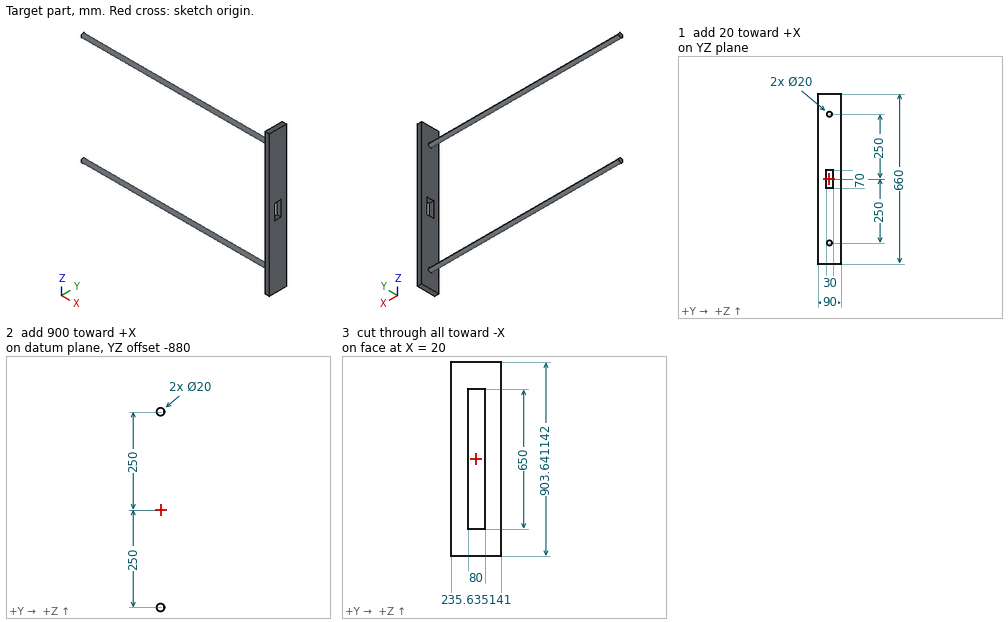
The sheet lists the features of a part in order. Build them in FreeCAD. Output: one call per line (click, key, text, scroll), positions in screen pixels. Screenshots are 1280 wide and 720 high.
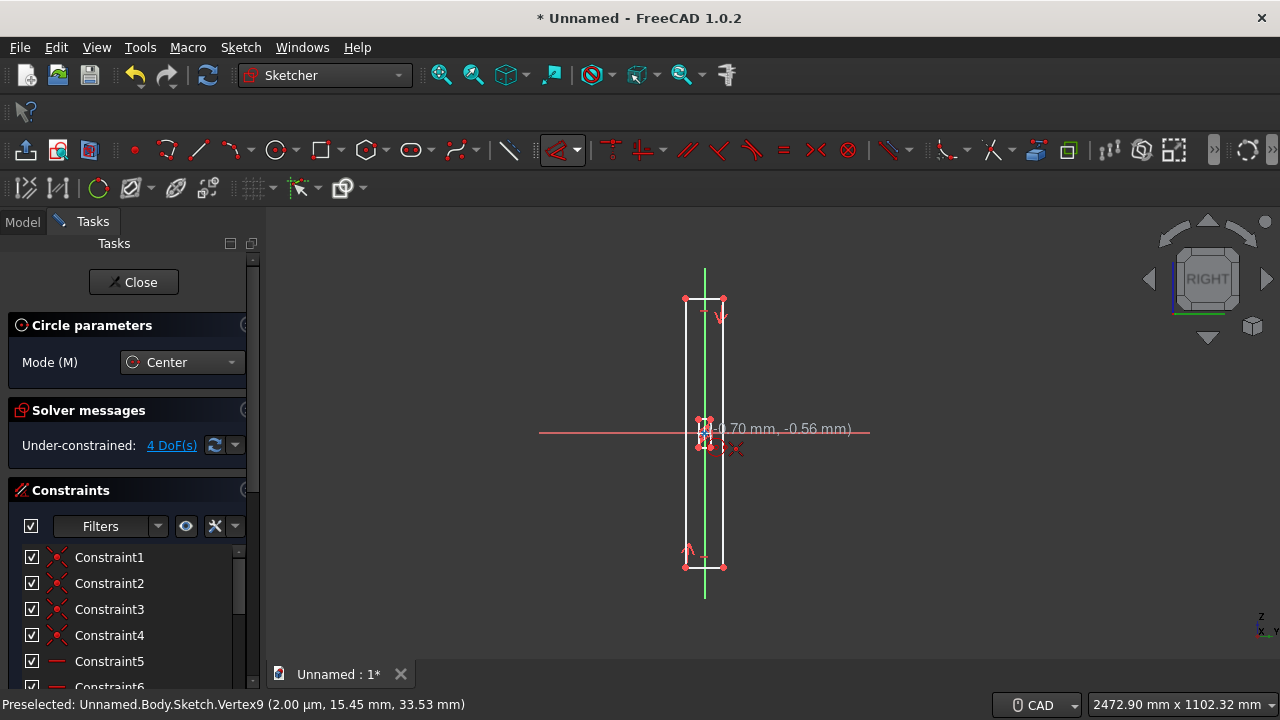
scroll(705, 331, up, 9)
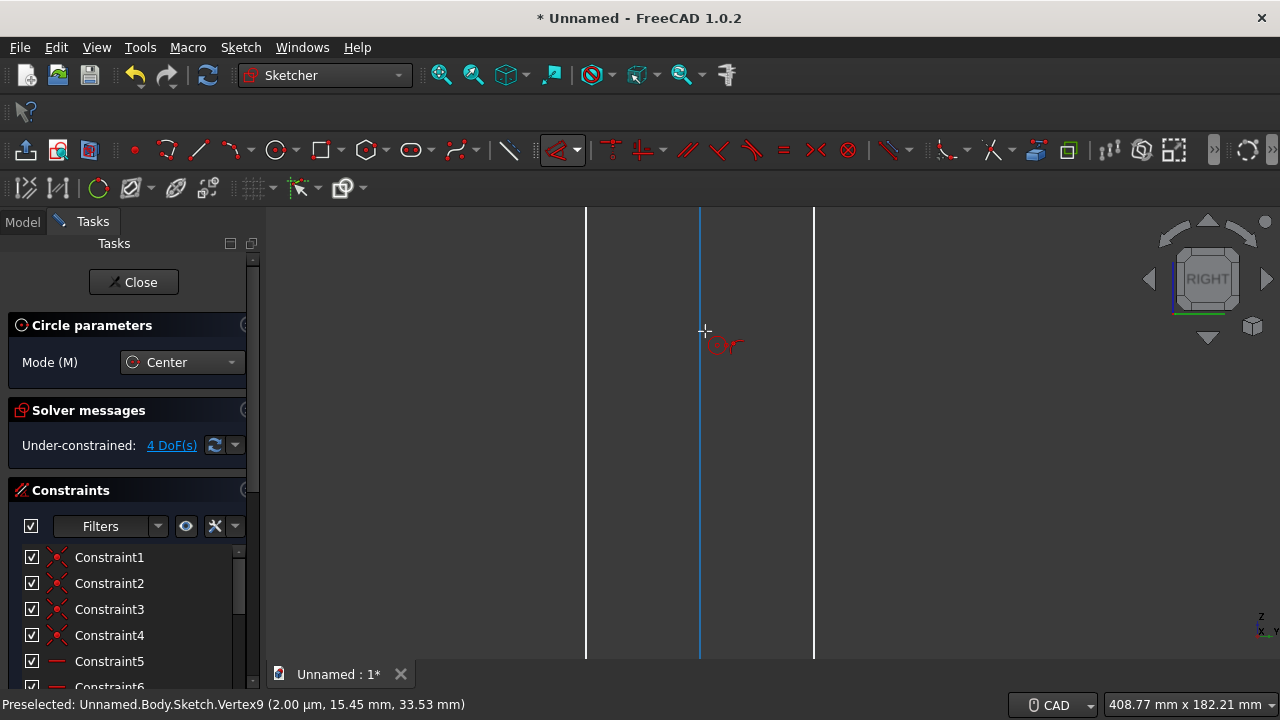
scroll(705, 331, down, 9)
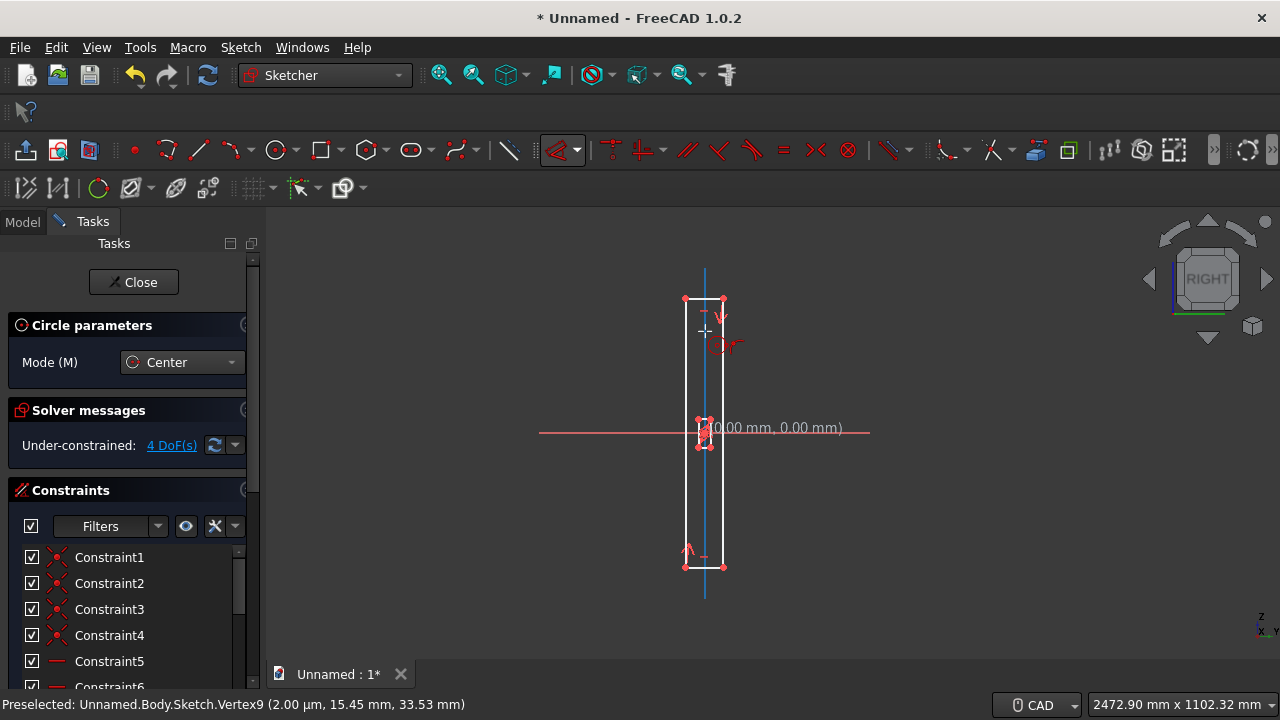
click(705, 331)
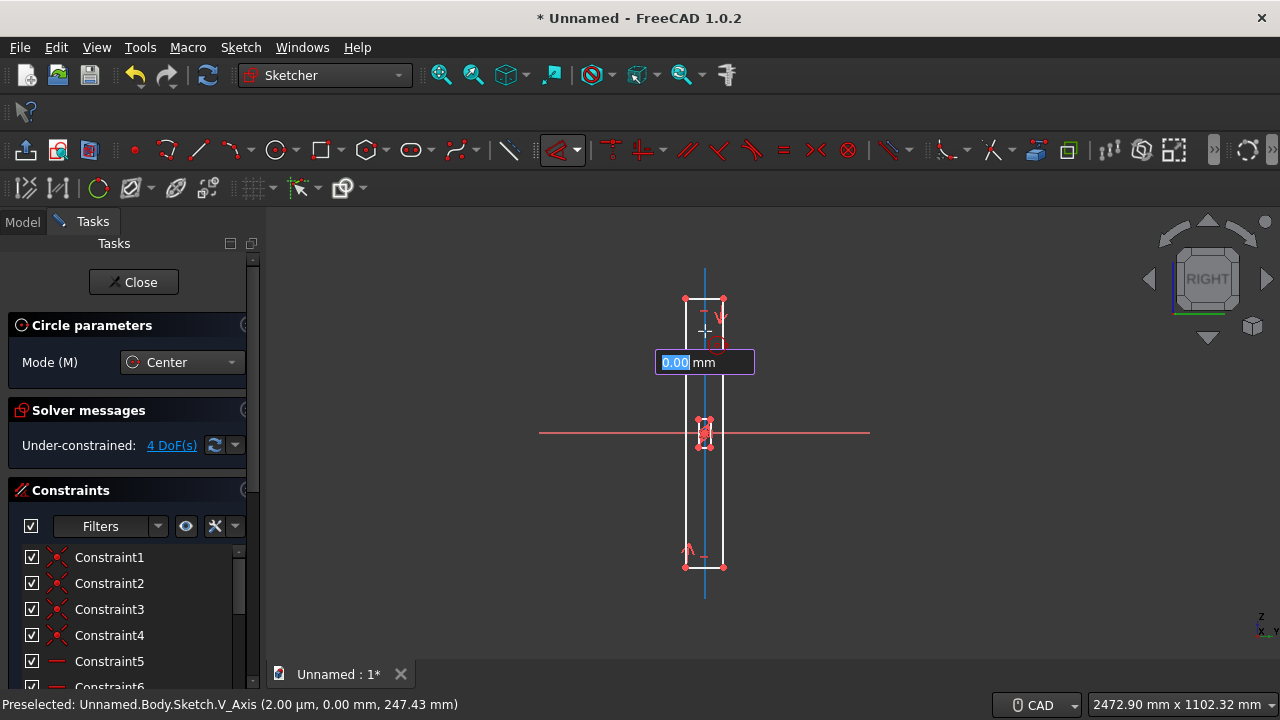
scroll(708, 330, up, 8)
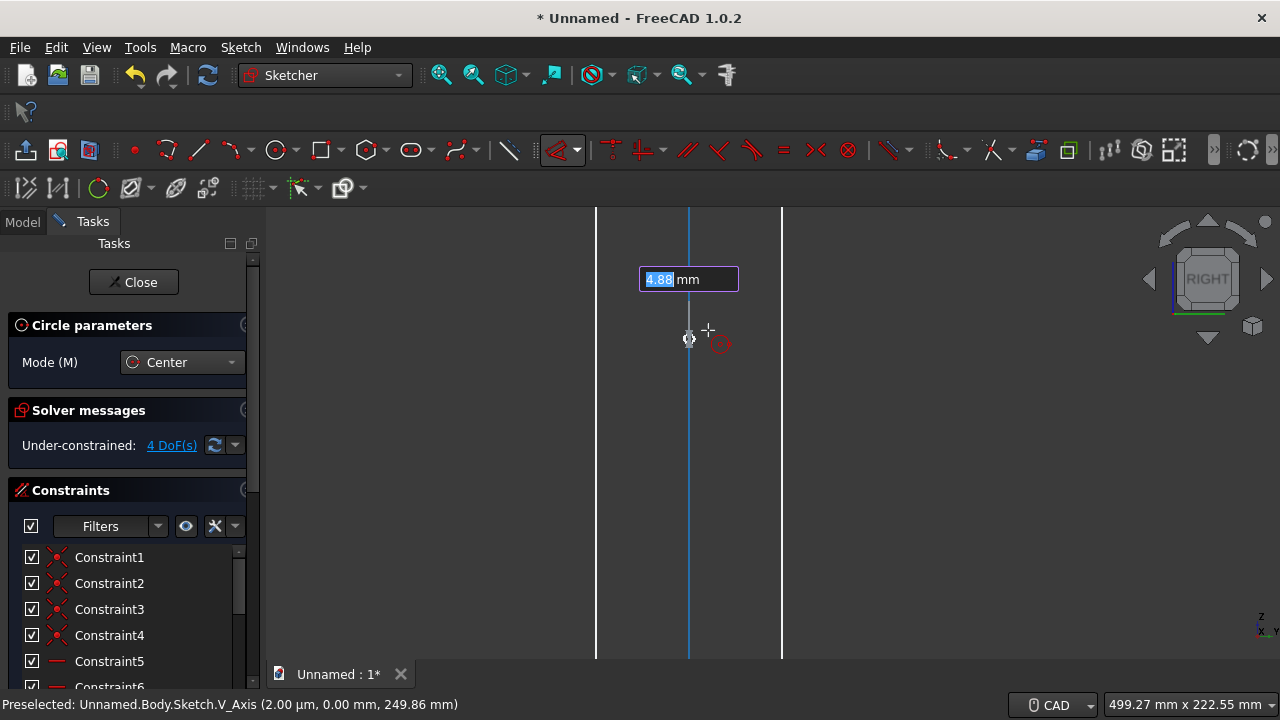
click(708, 327)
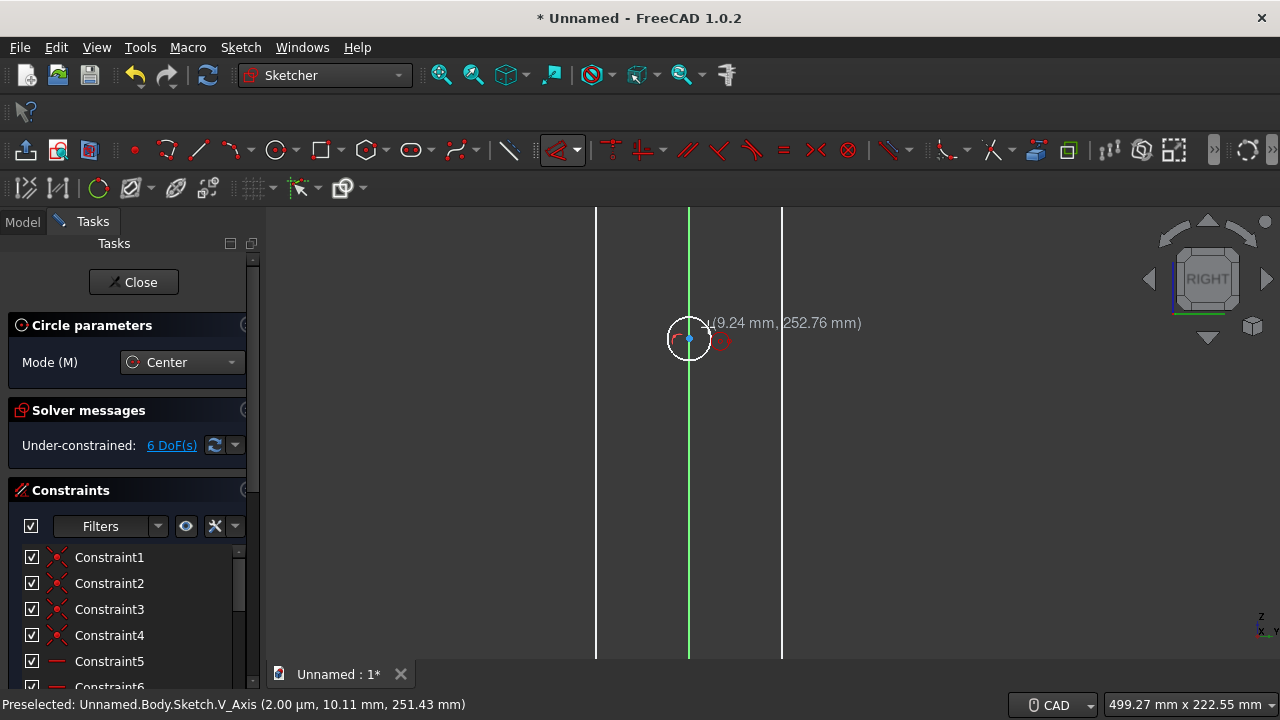
scroll(708, 330, down, 8)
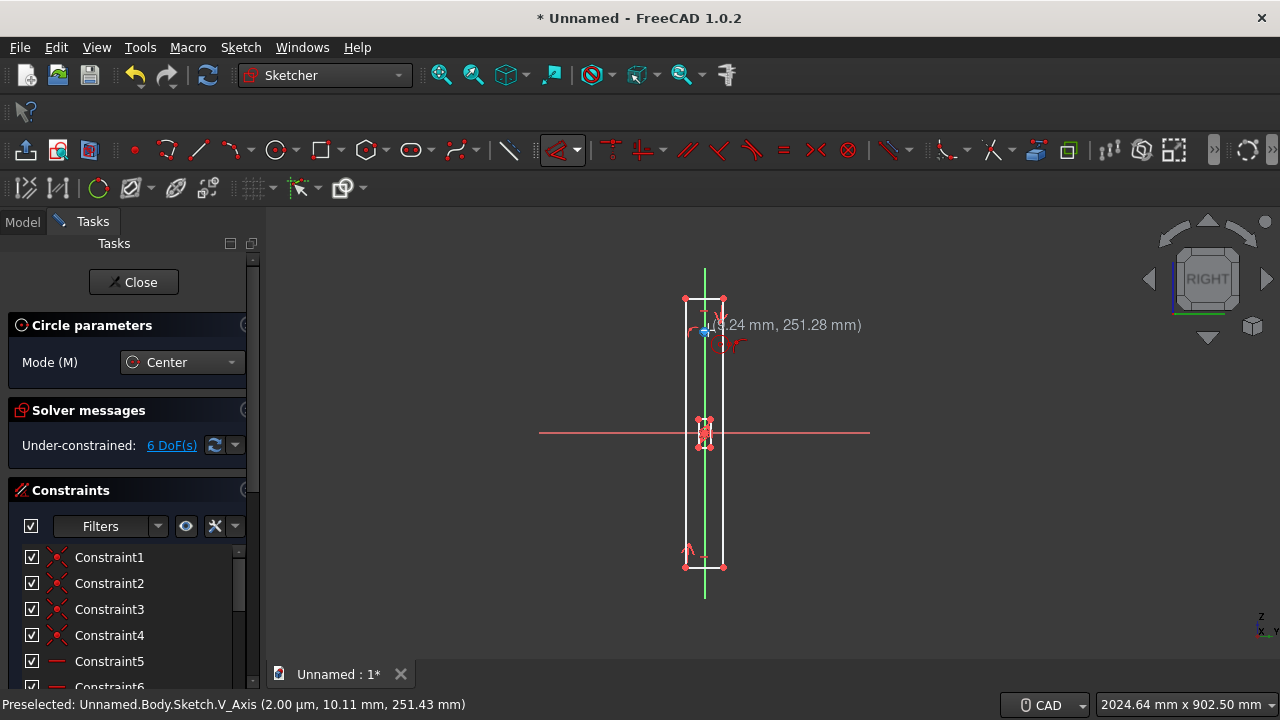
scroll(705, 536, up, 9)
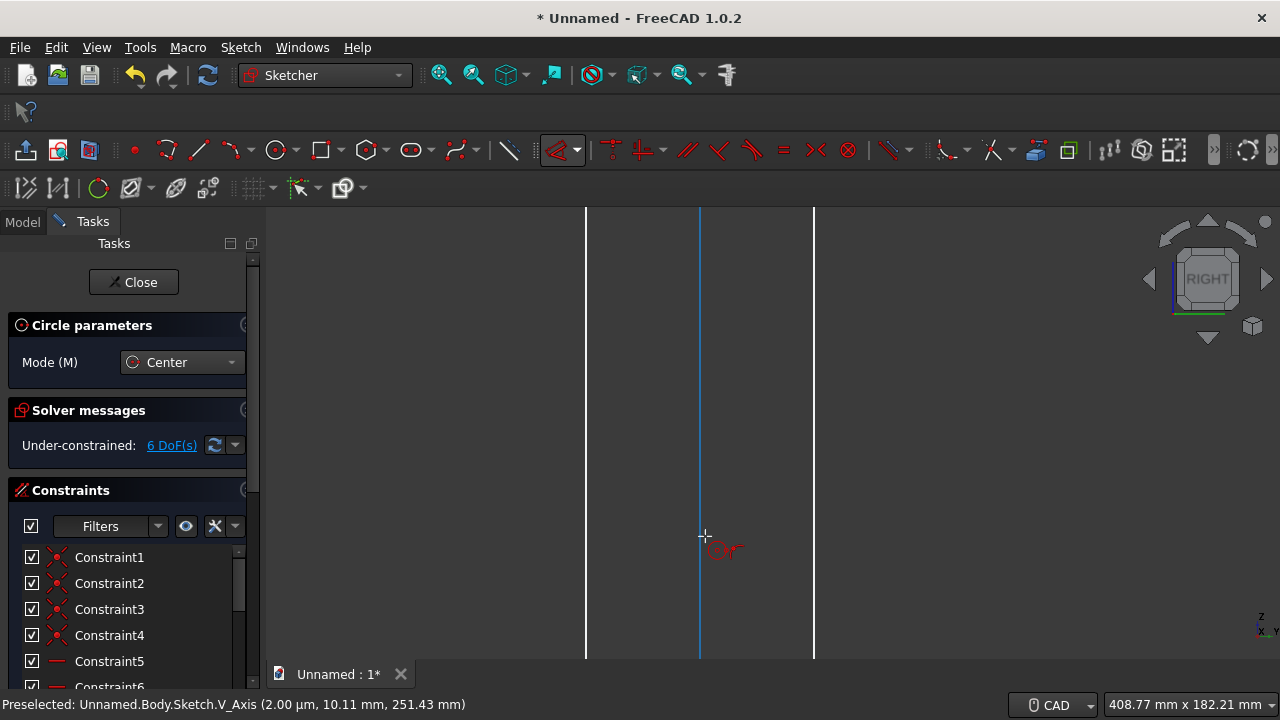
scroll(705, 536, down, 9)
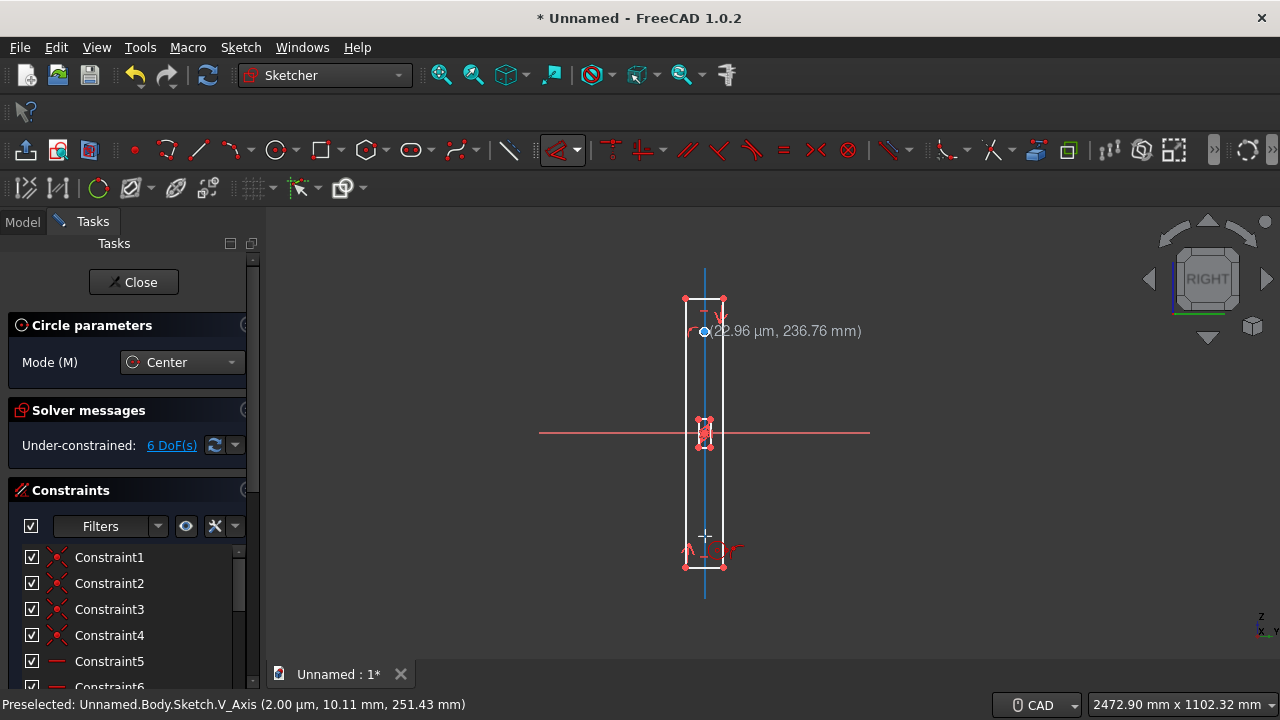
click(705, 536)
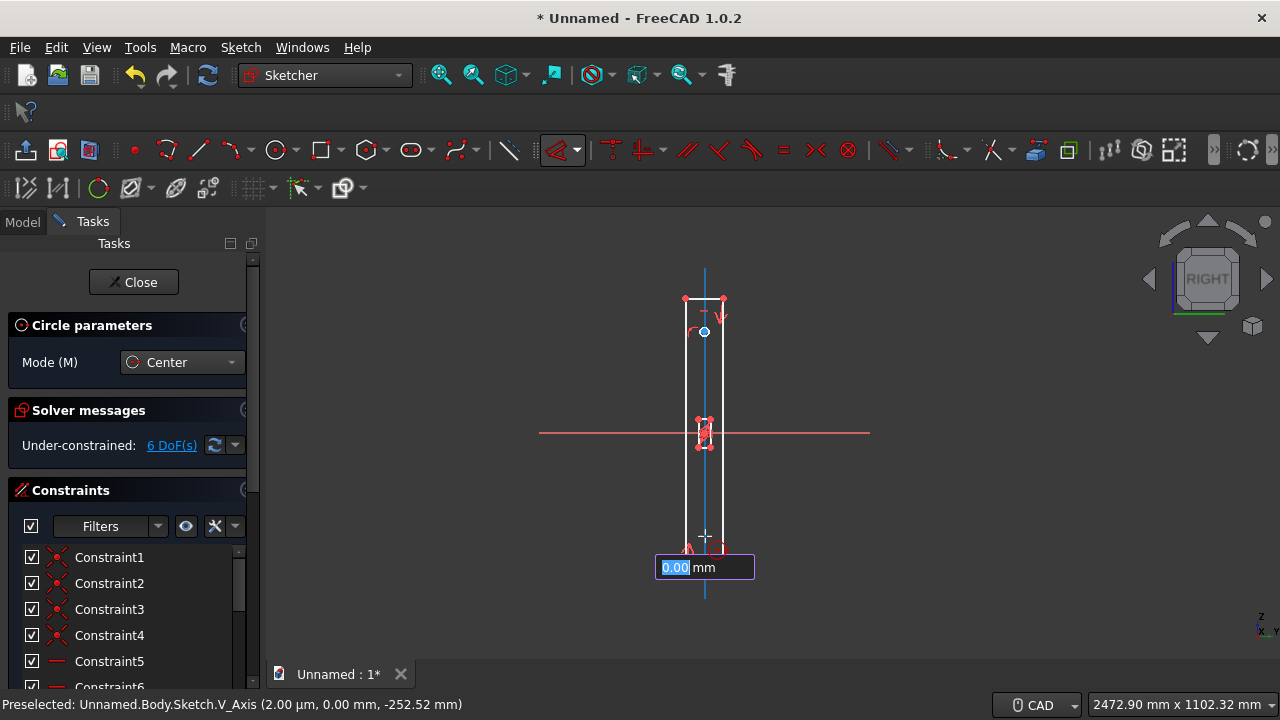
scroll(708, 535, up, 8)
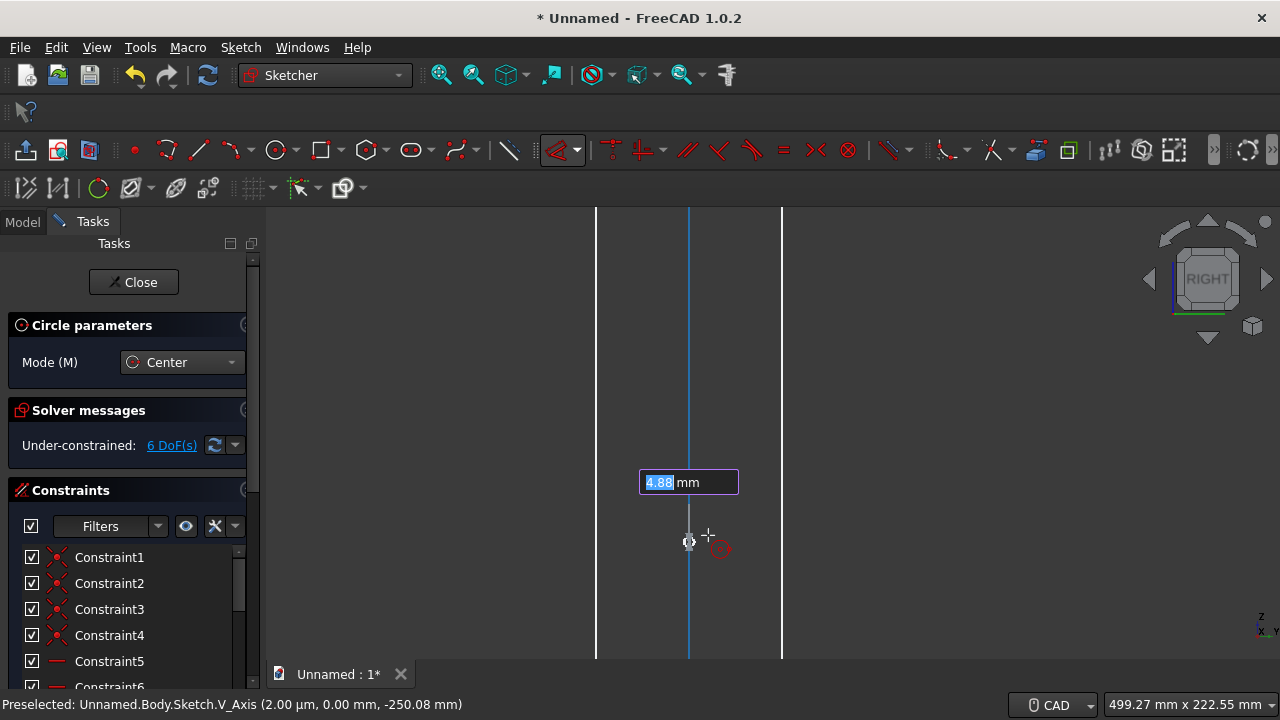
click(708, 530)
key(Escape)